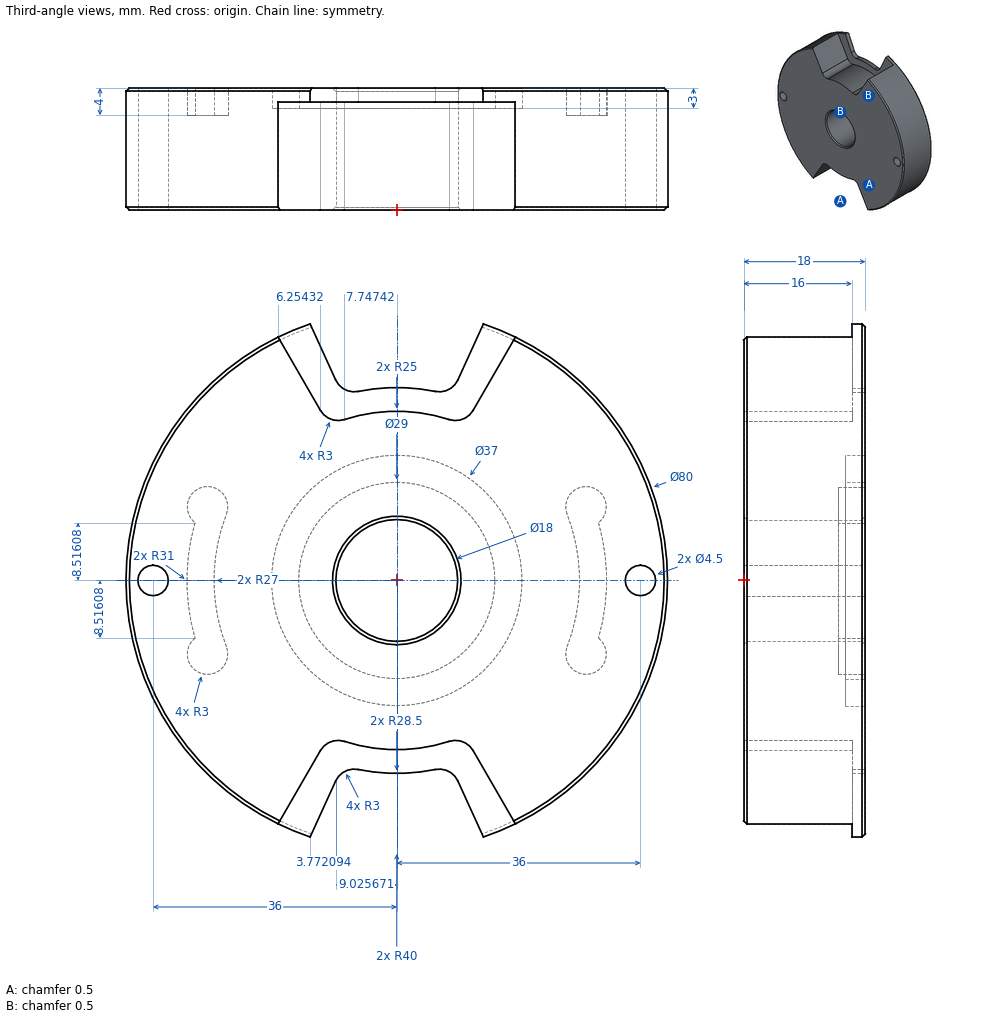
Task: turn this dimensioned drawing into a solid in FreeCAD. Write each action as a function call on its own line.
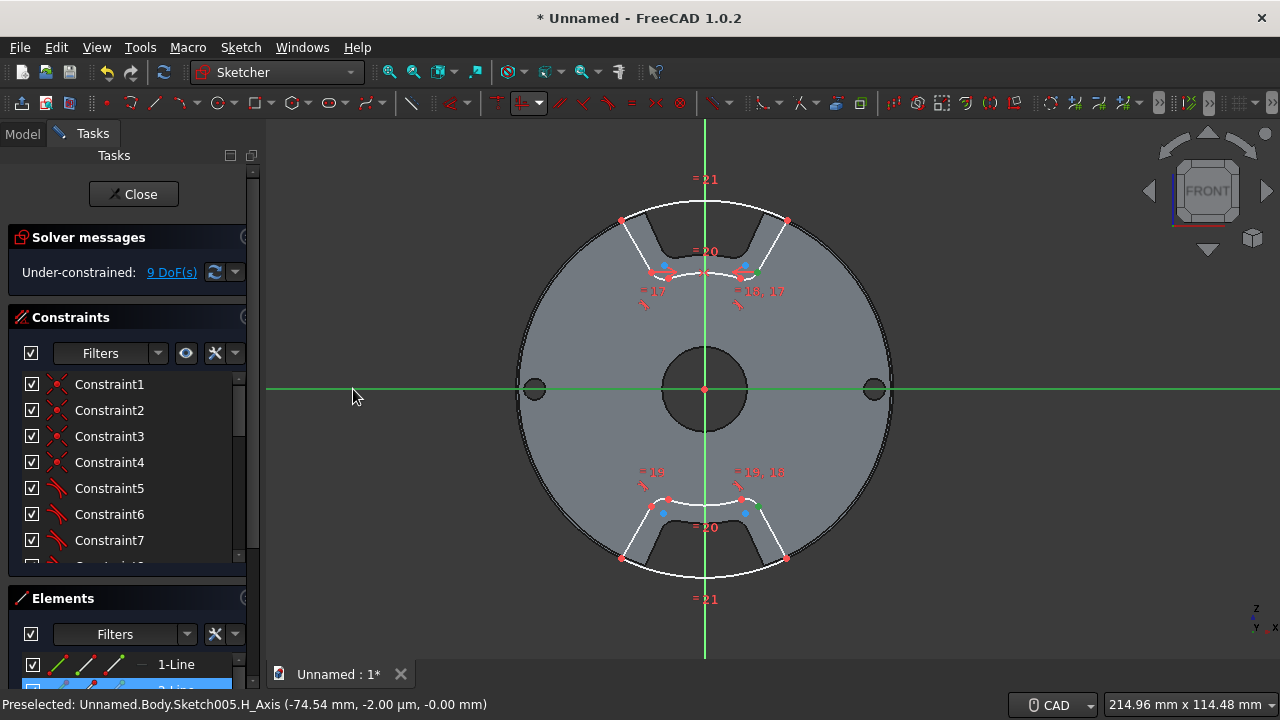
click(656, 104)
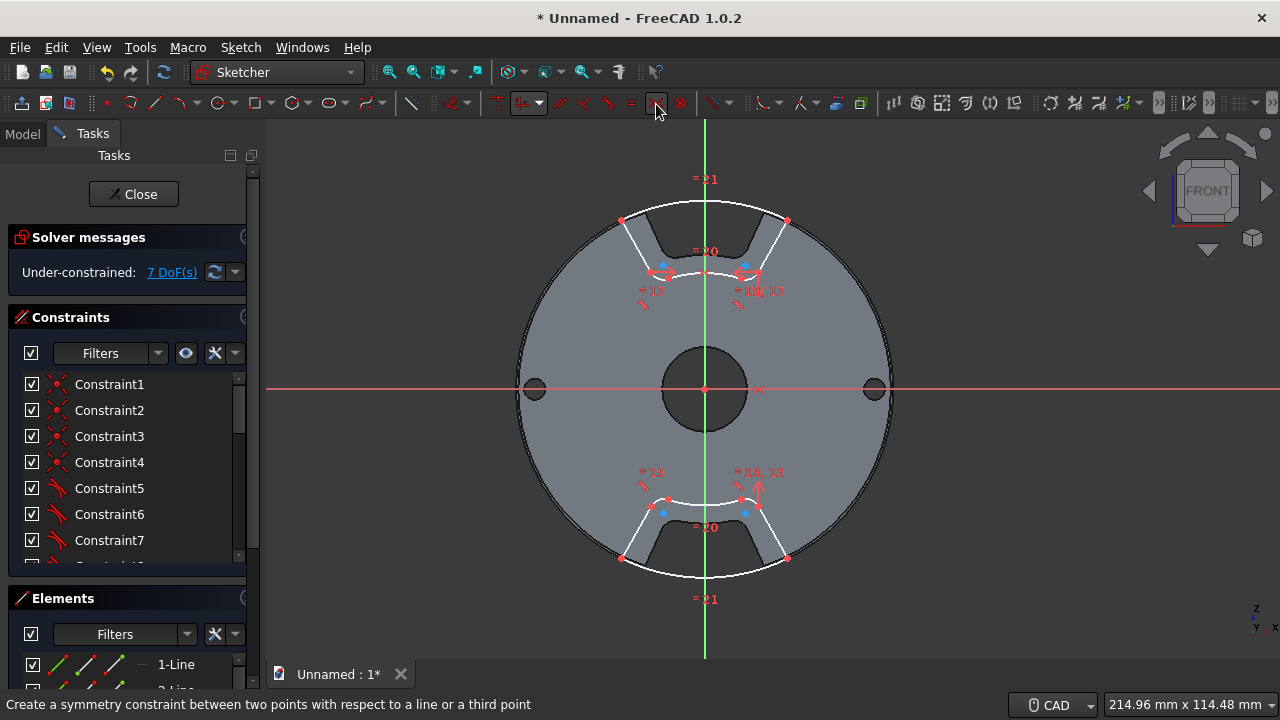
click(651, 272)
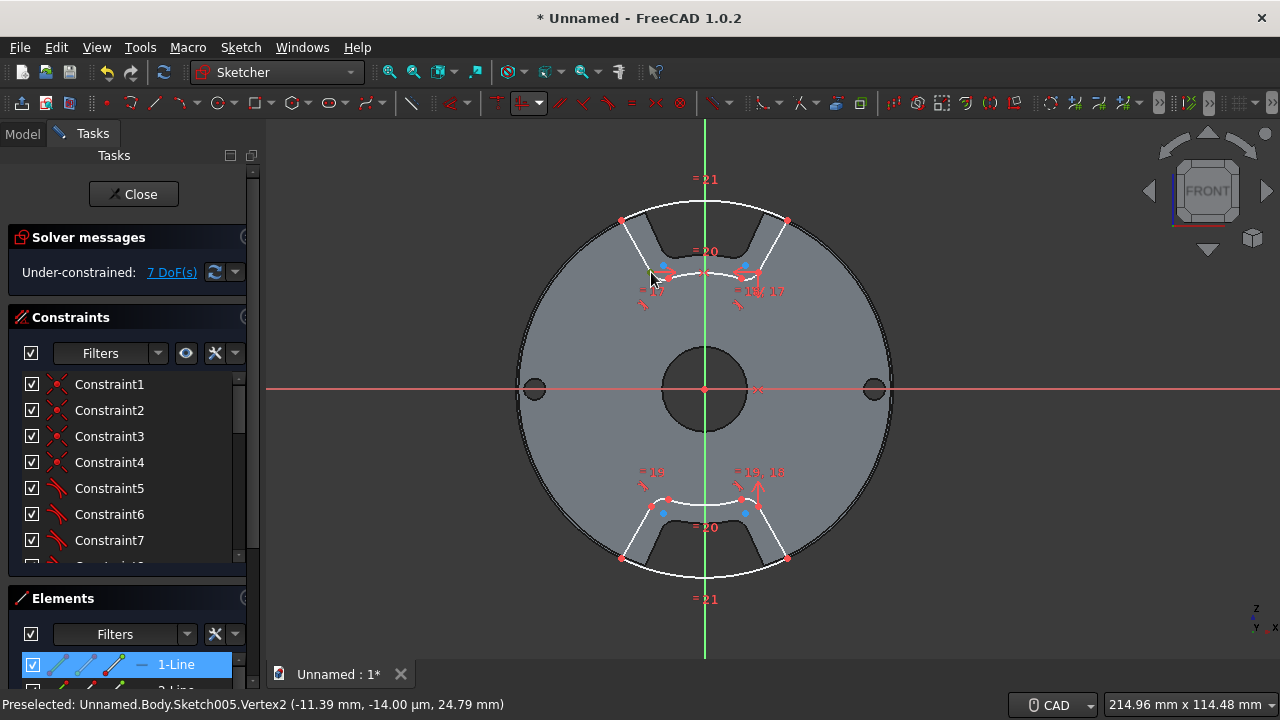
click(651, 506)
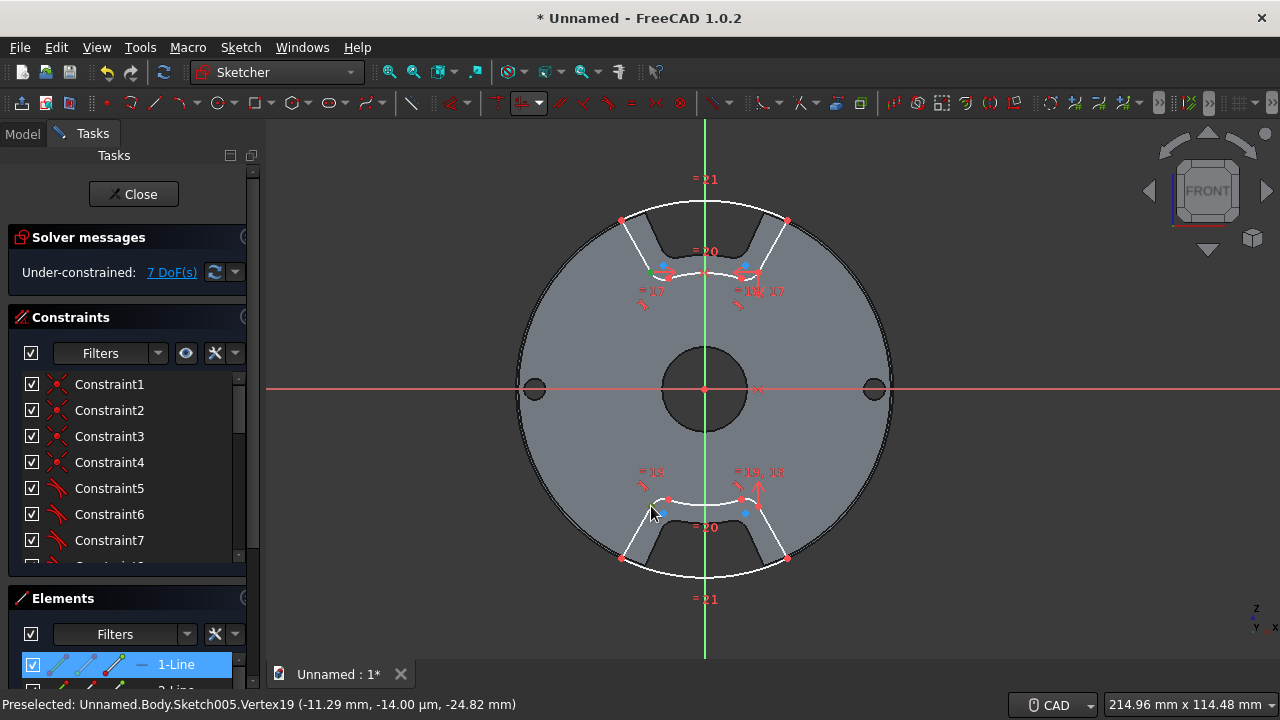
click(353, 389)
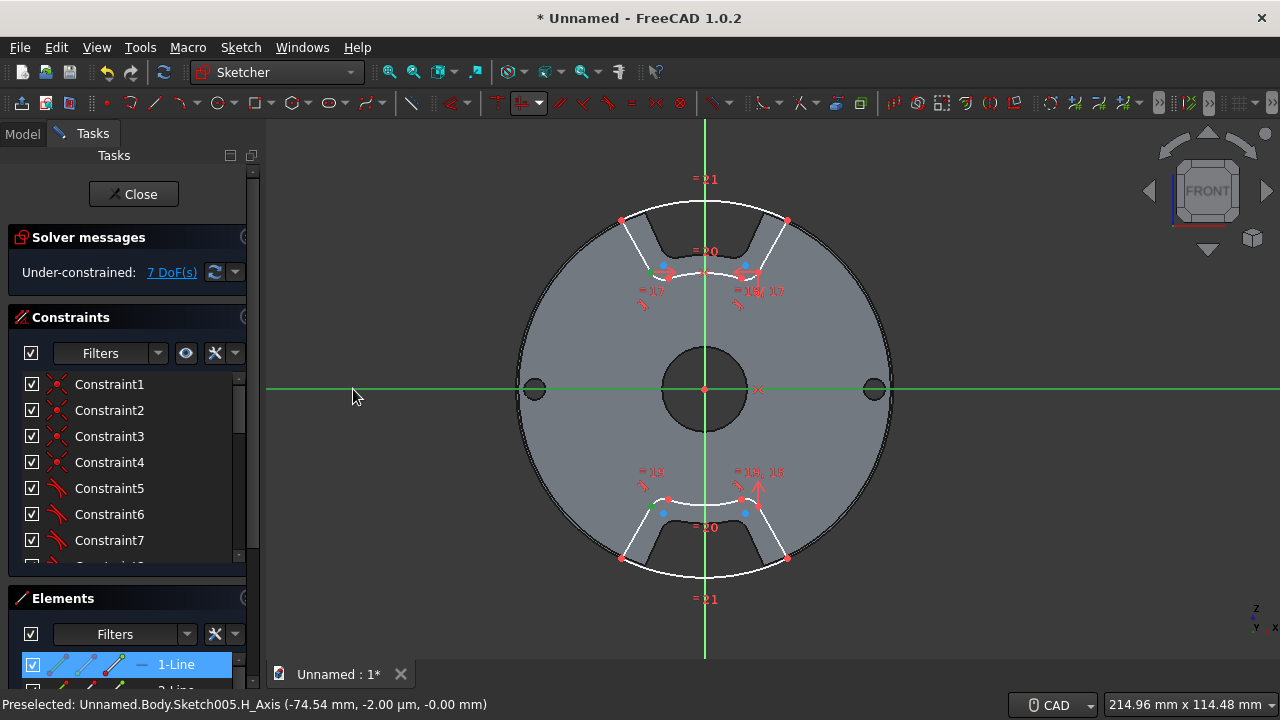
click(656, 104)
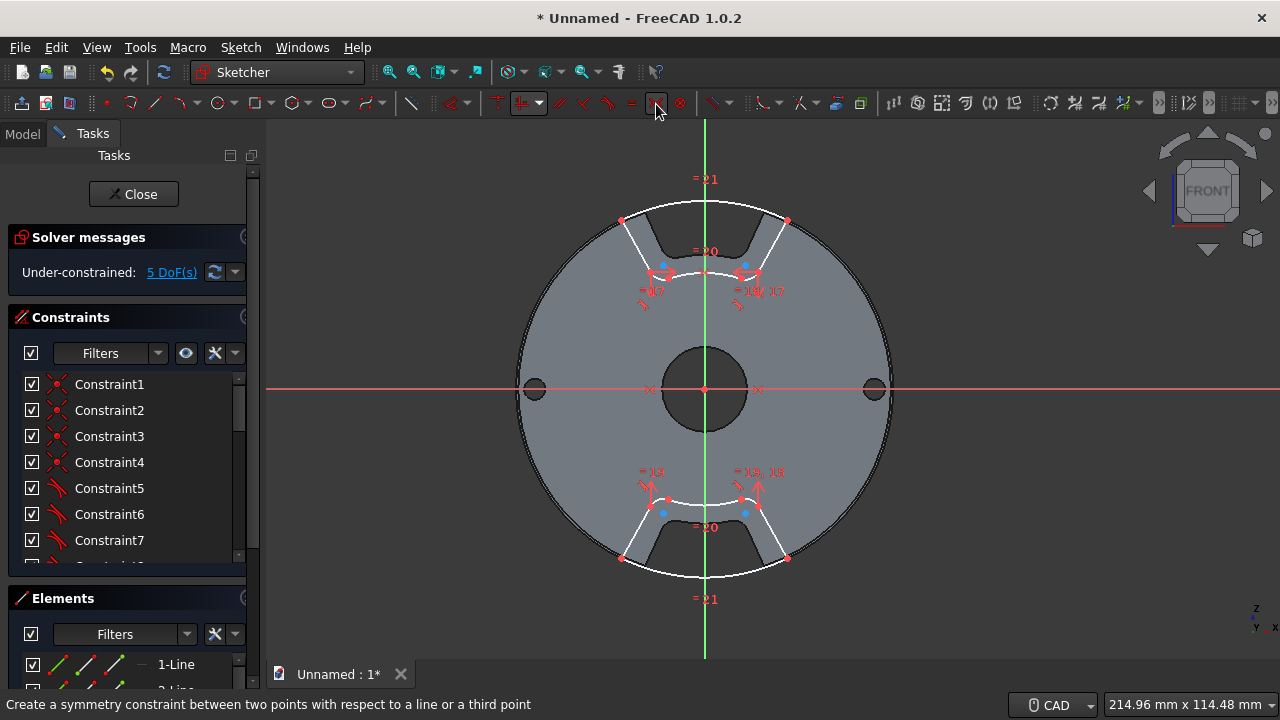
click(450, 104)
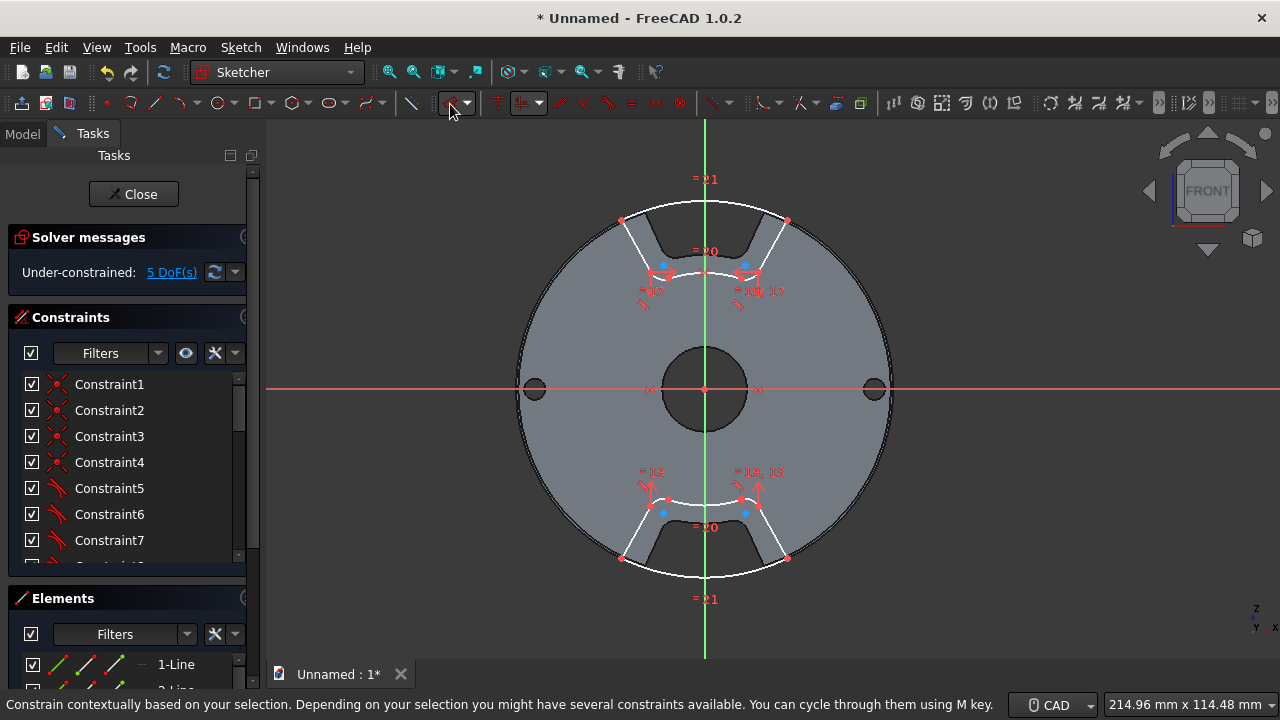
scroll(658, 279, up, 6)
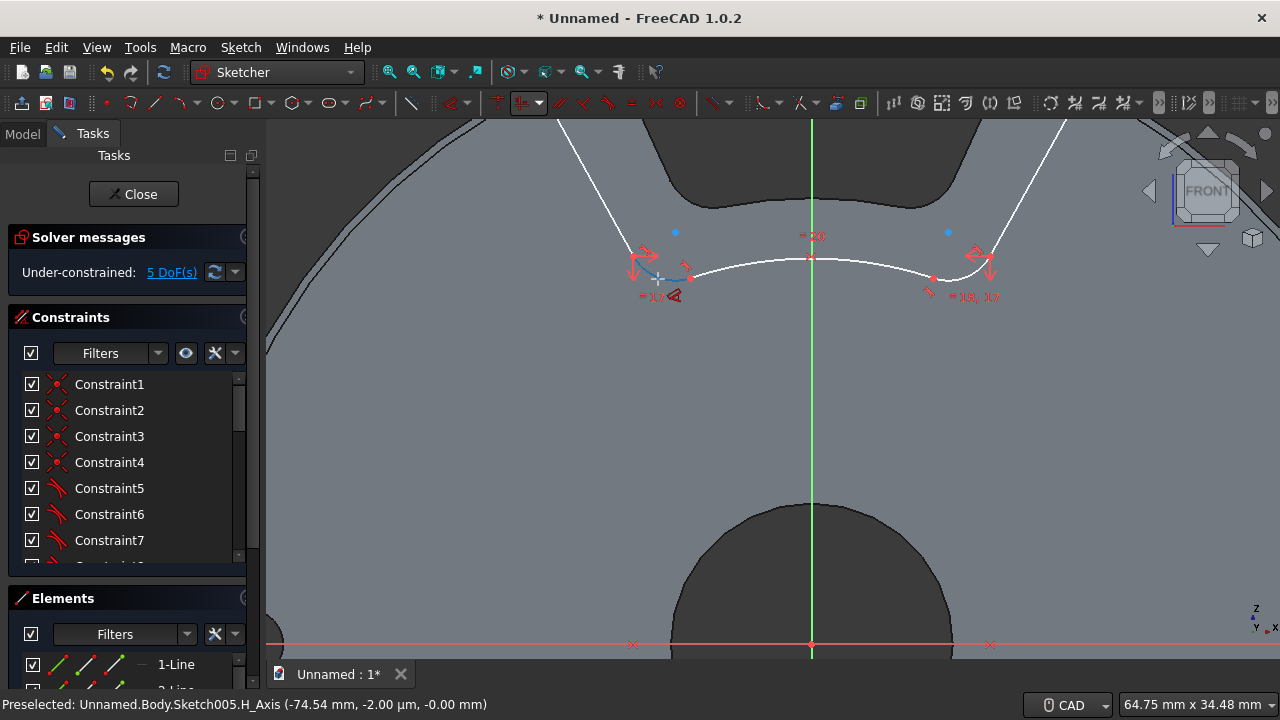
click(658, 277)
click(646, 307)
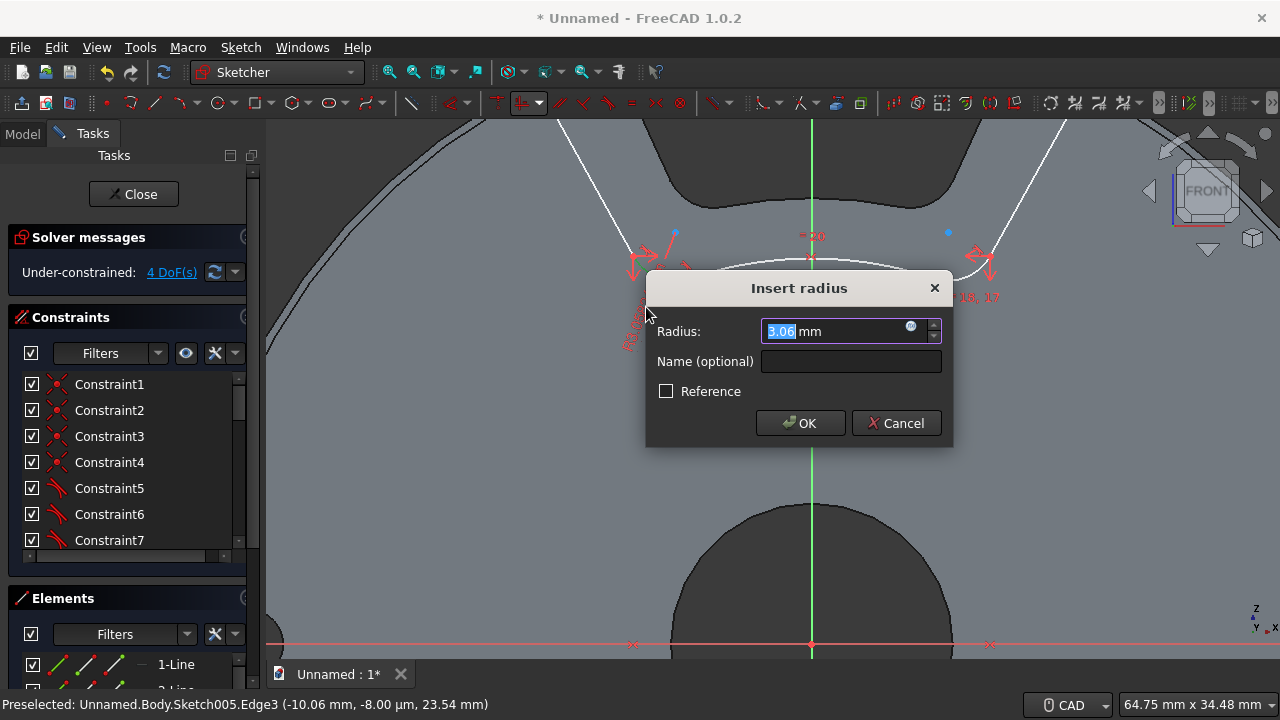
text(3)
key(Return)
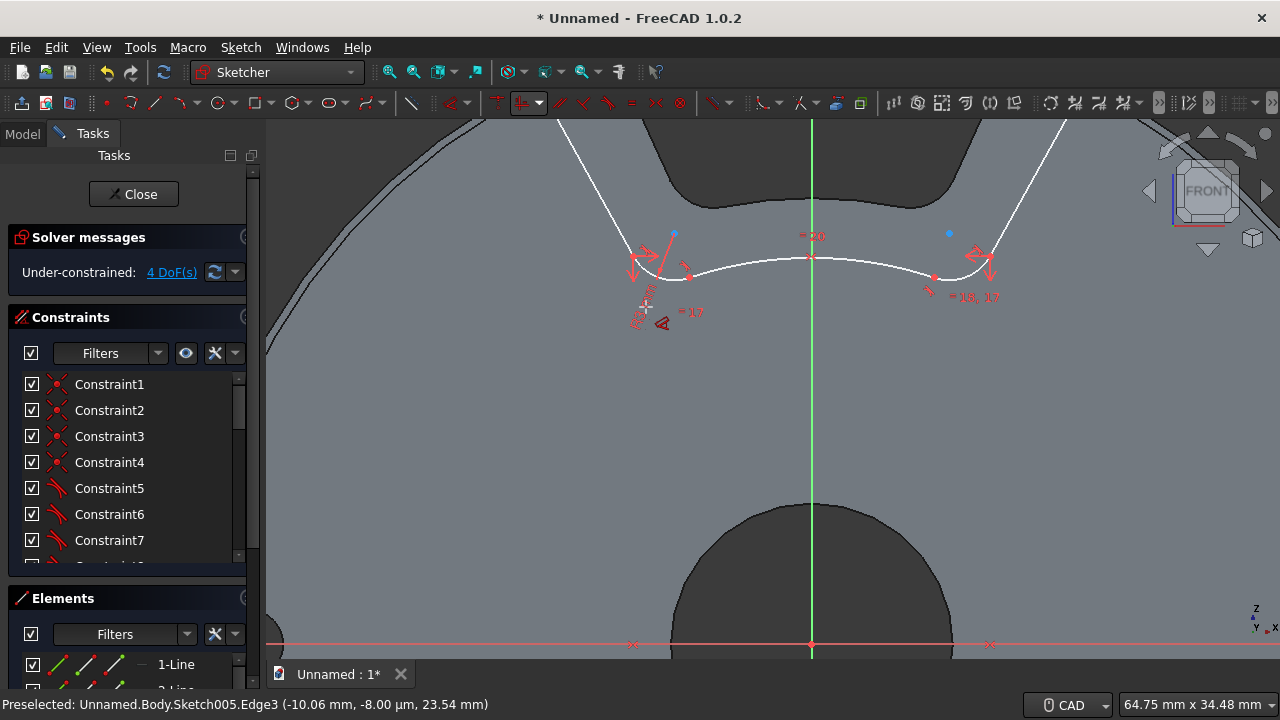
click(862, 261)
click(866, 229)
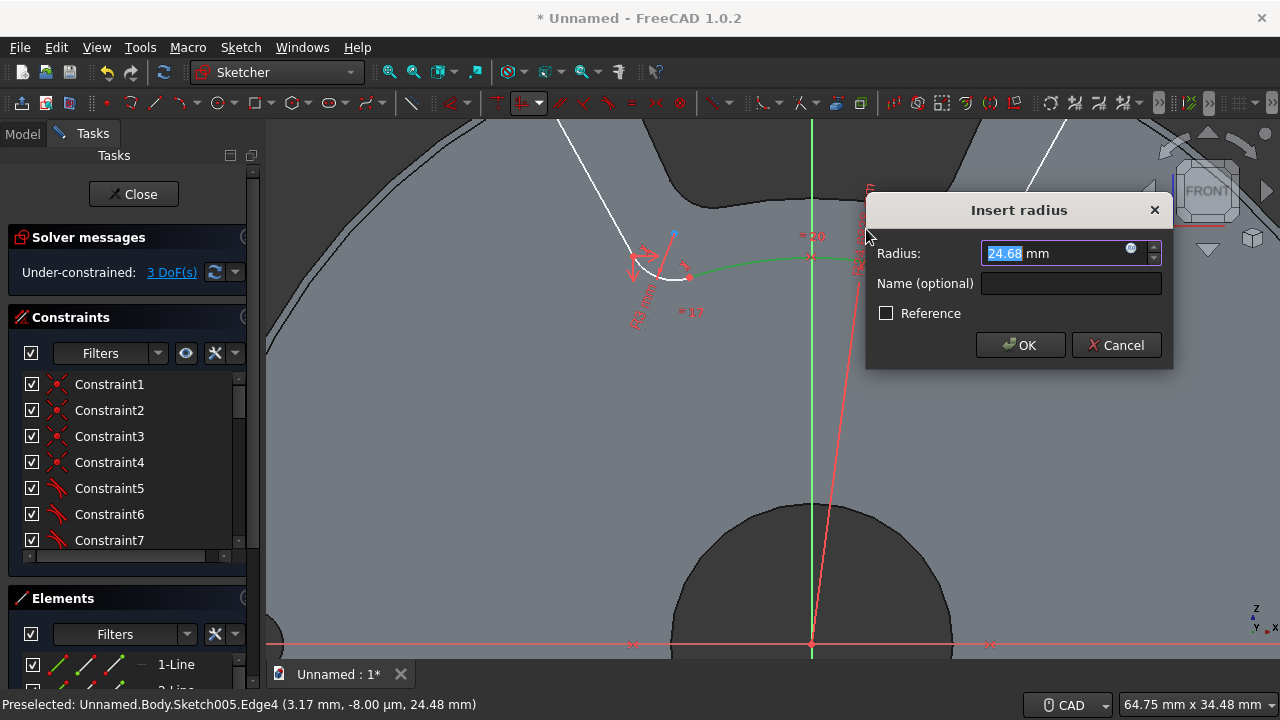
text(25)
key(Return)